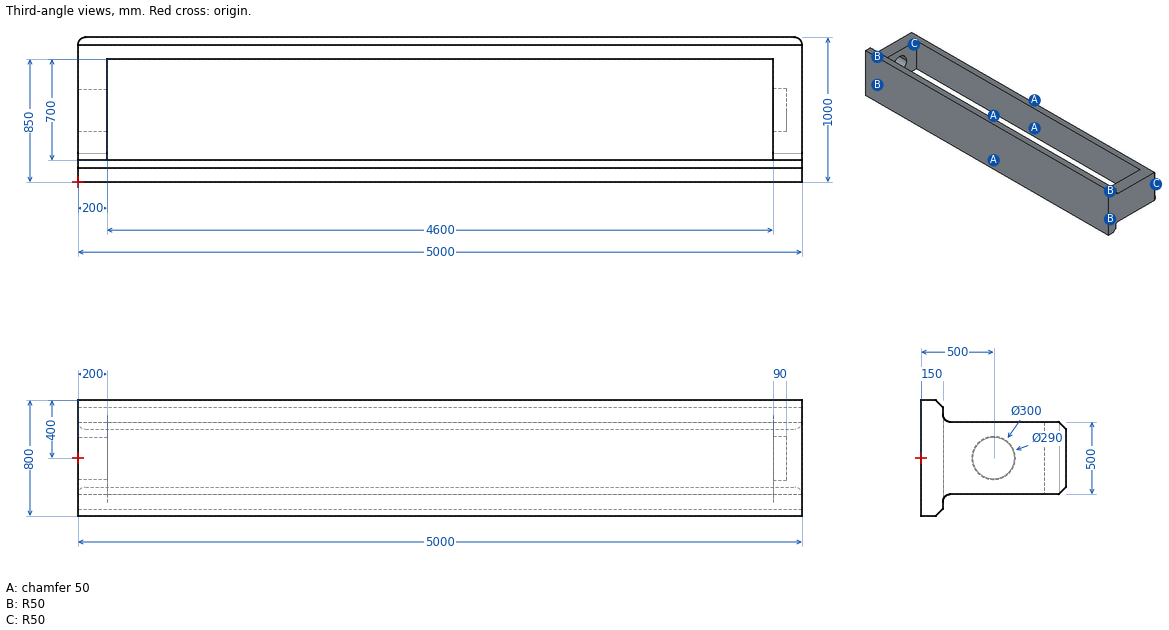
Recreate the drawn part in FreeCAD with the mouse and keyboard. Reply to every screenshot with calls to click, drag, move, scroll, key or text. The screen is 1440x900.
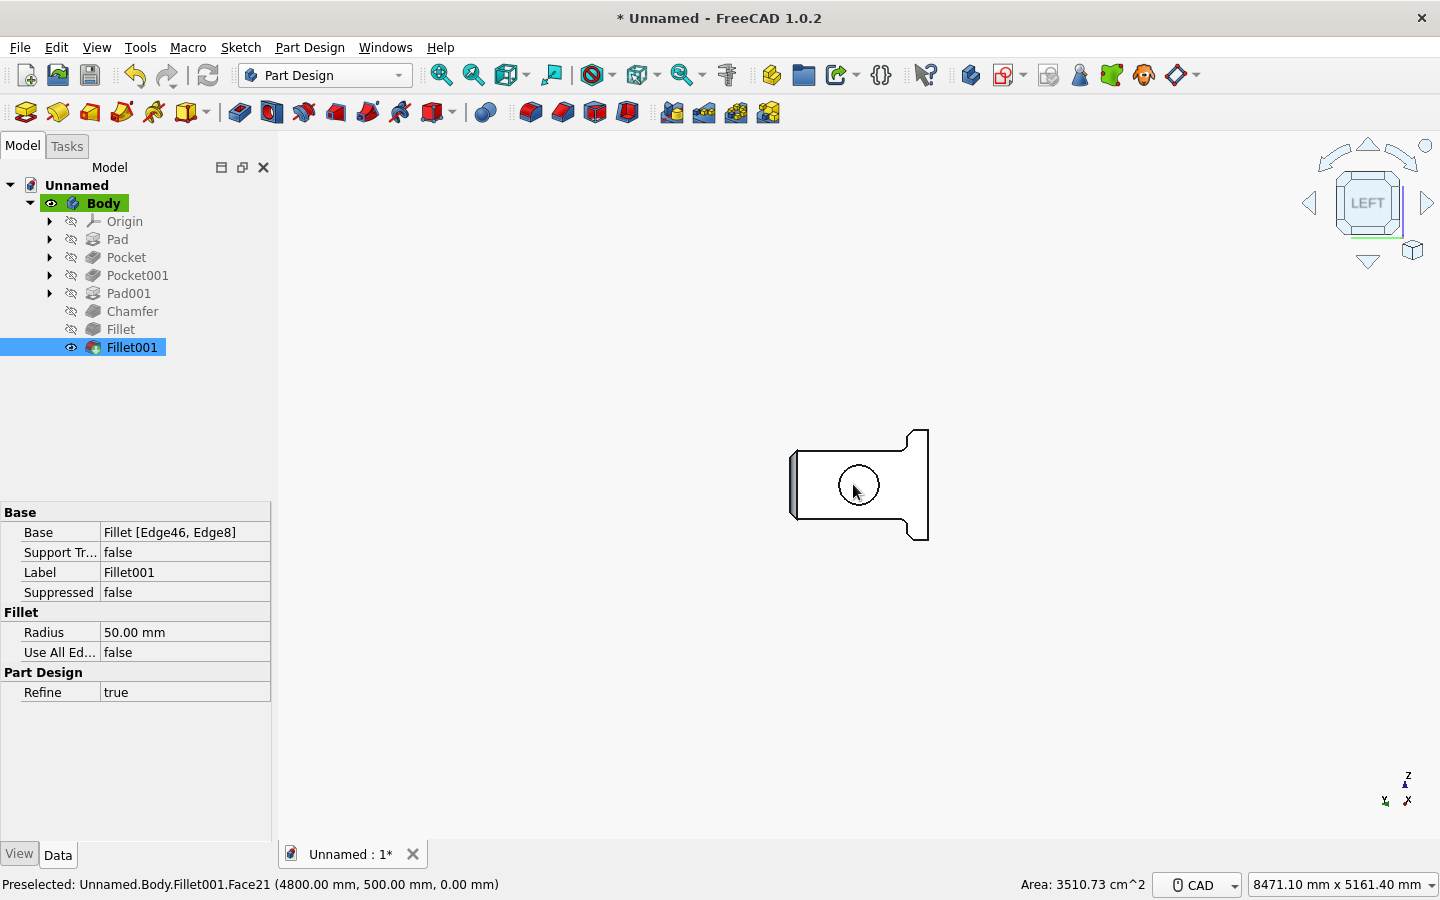
click(1004, 76)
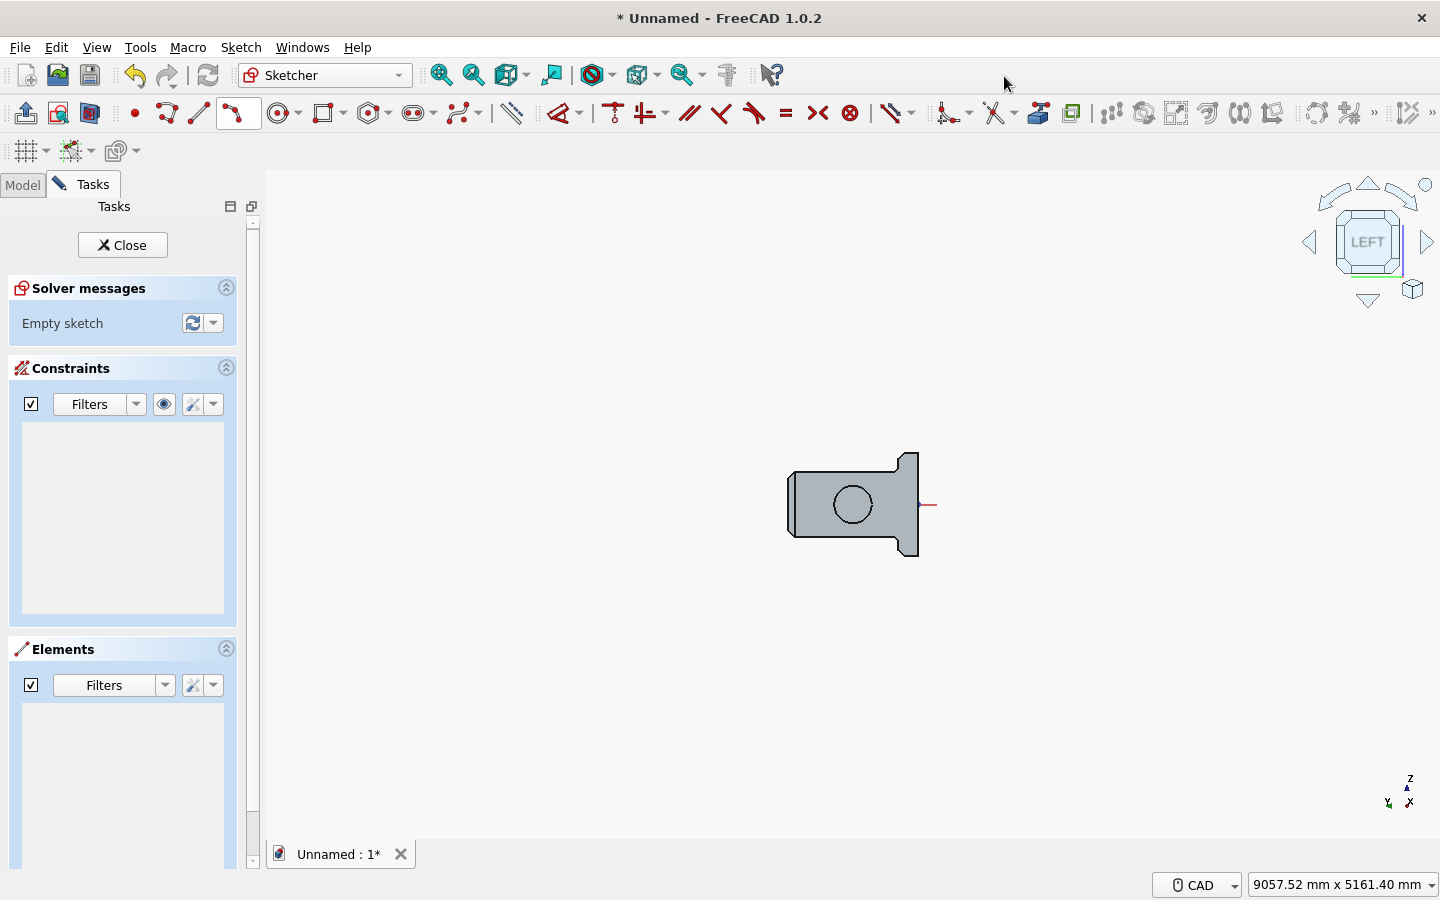
key(q)
key(s)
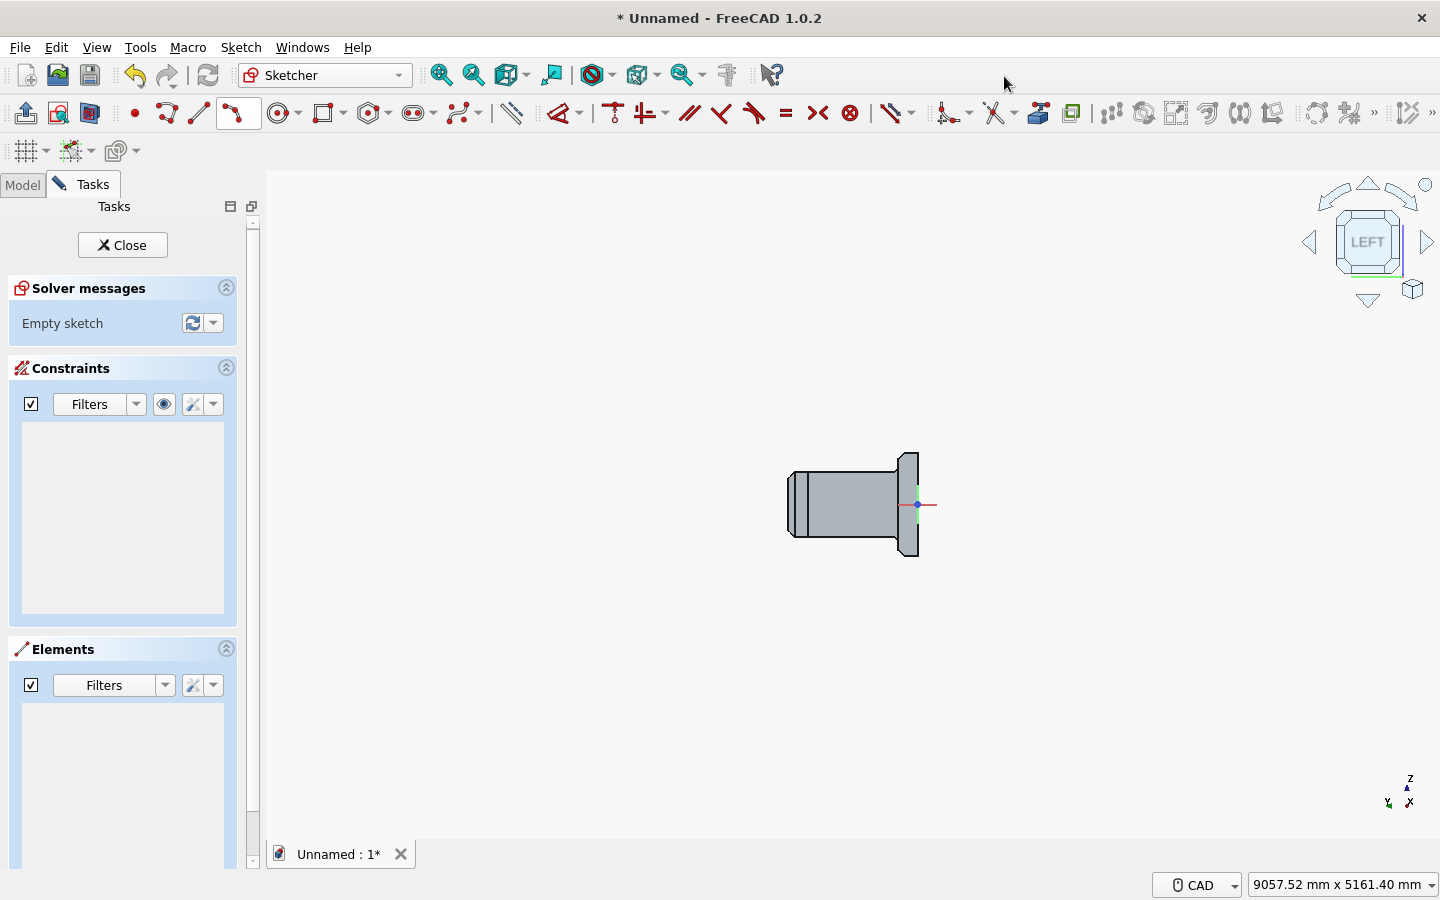
scroll(887, 504, up, 11)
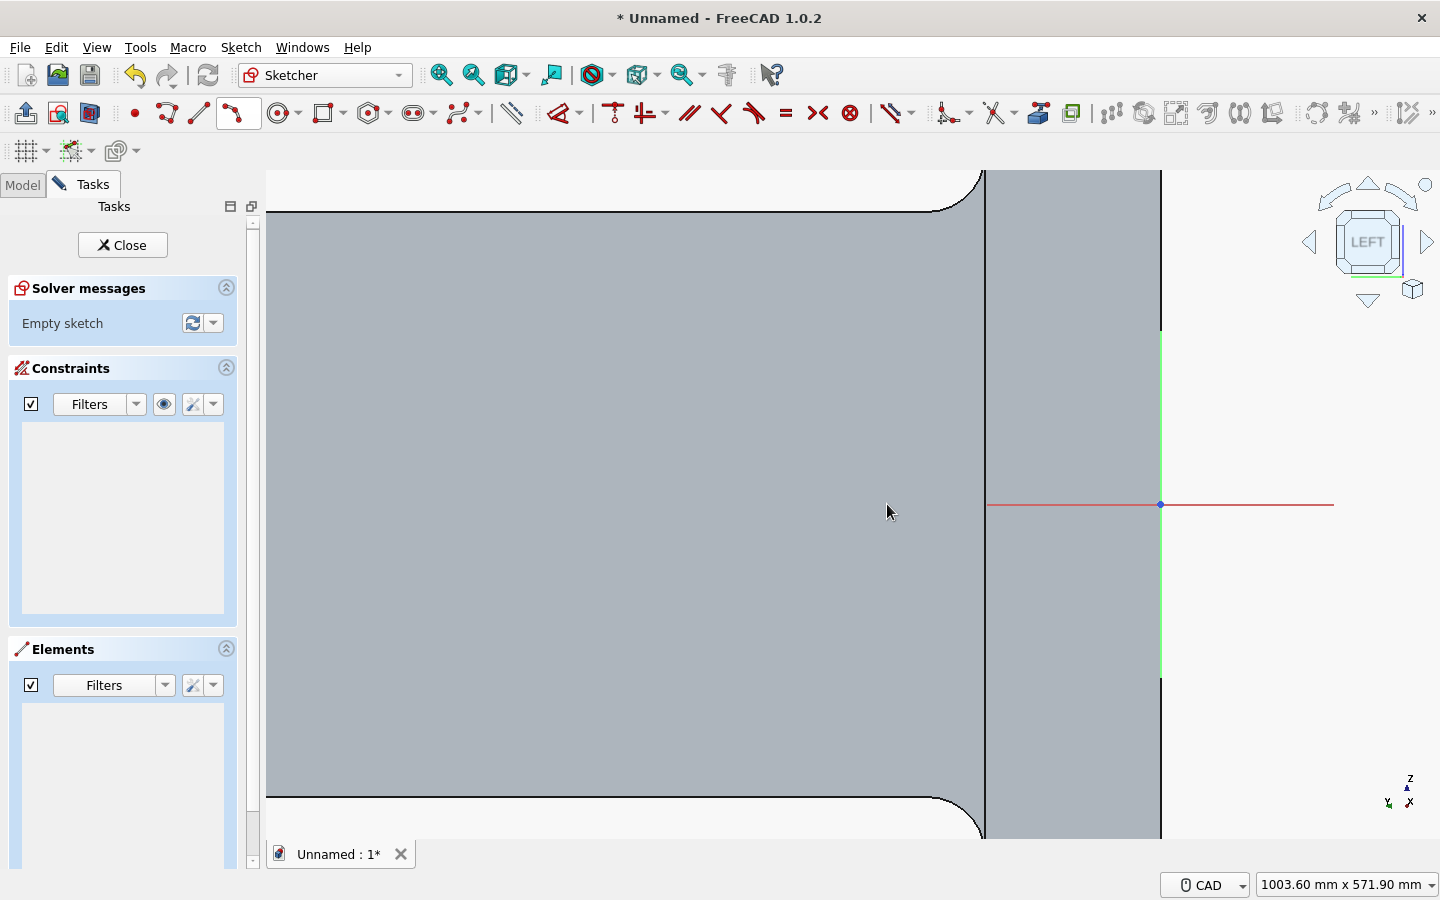
key(g)
key(c)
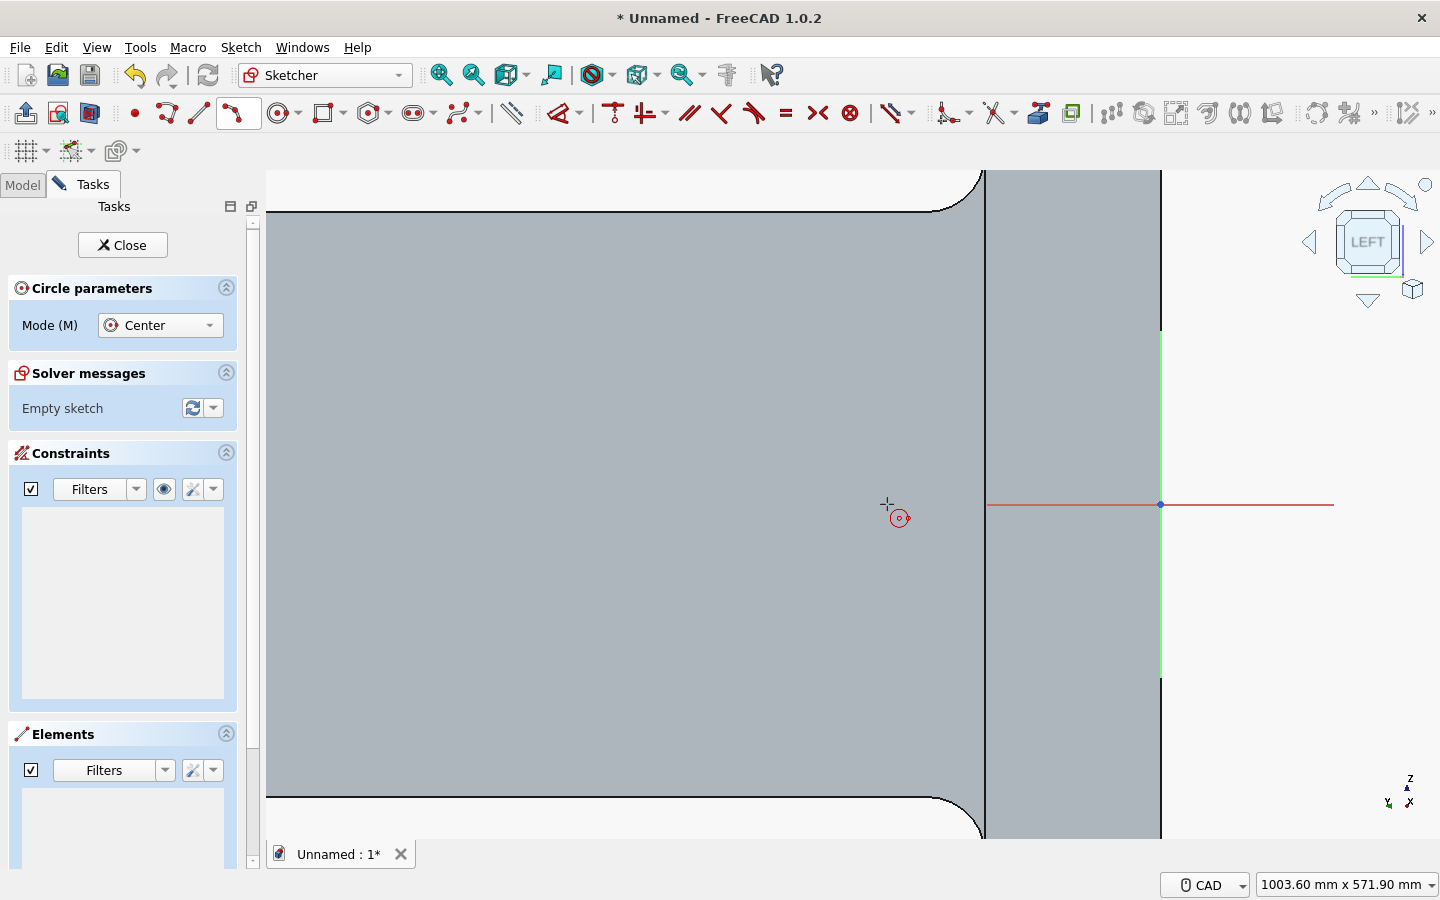
click(576, 504)
click(700, 380)
key(Escape)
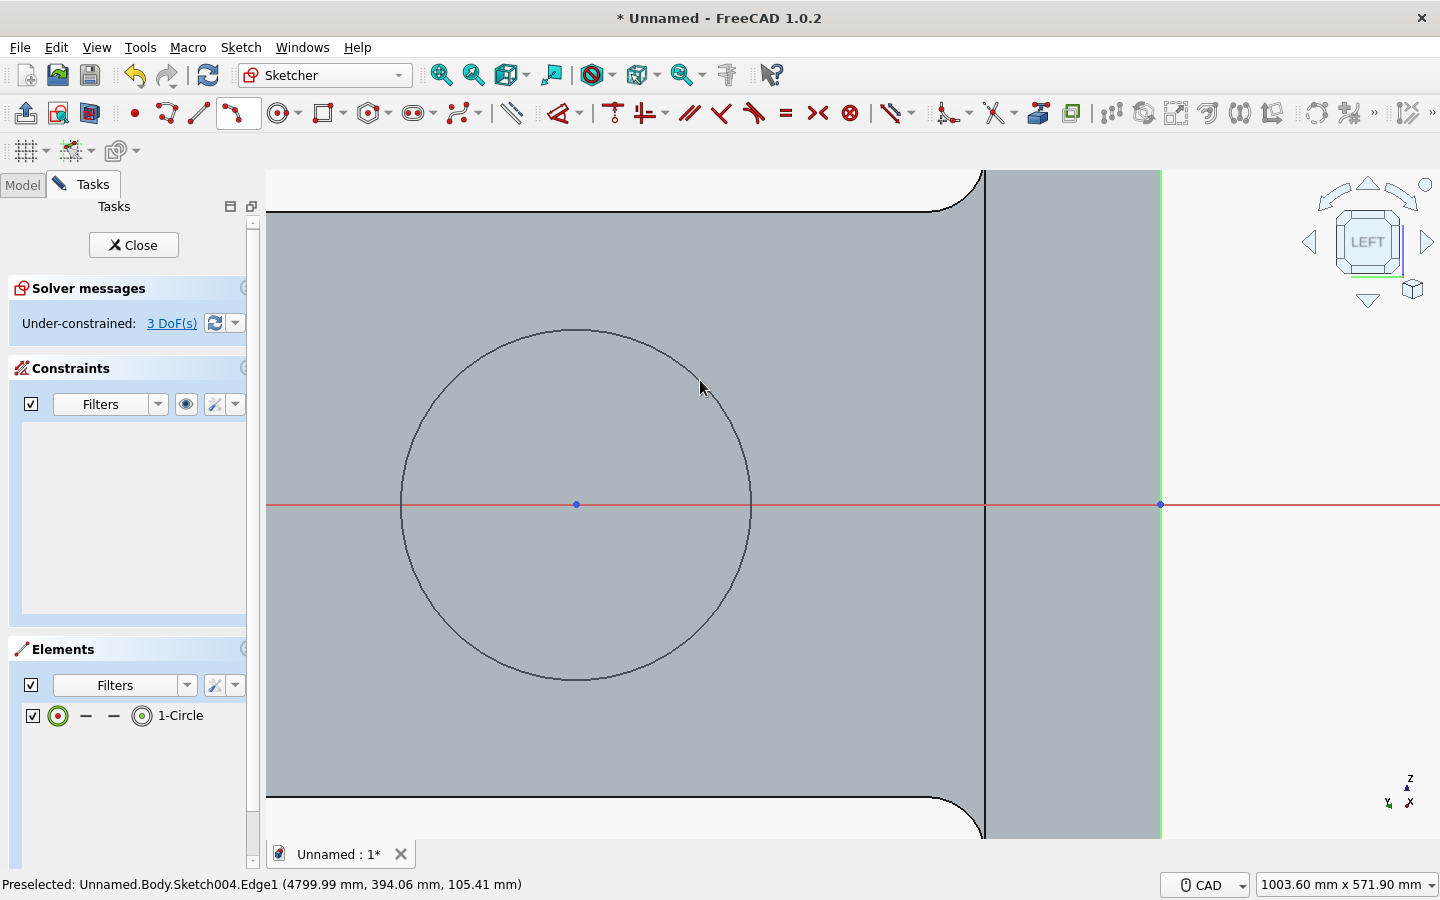
click(576, 505)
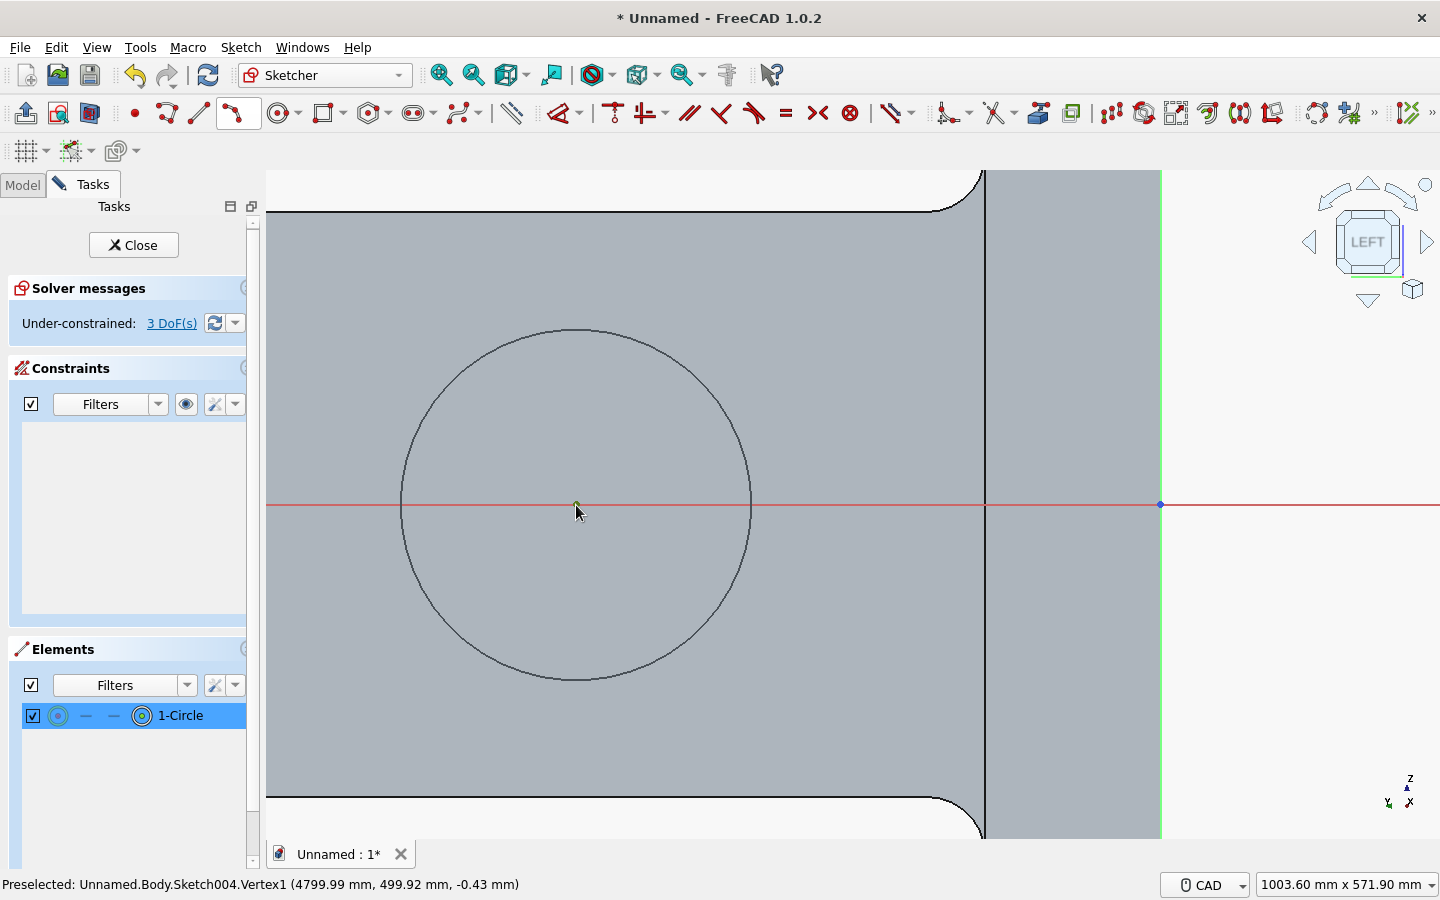
click(364, 504)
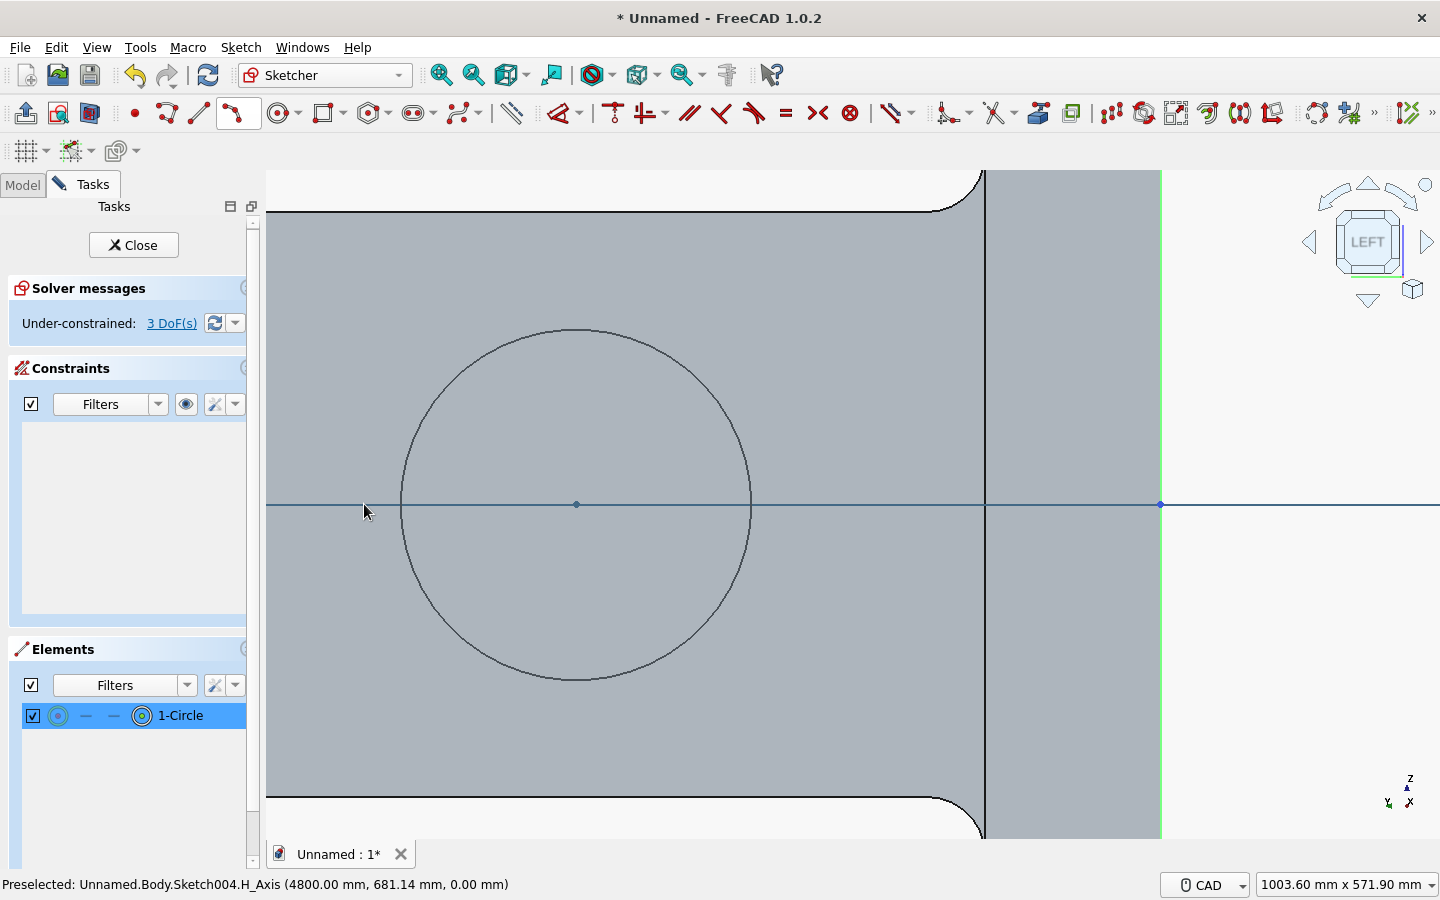
key(c)